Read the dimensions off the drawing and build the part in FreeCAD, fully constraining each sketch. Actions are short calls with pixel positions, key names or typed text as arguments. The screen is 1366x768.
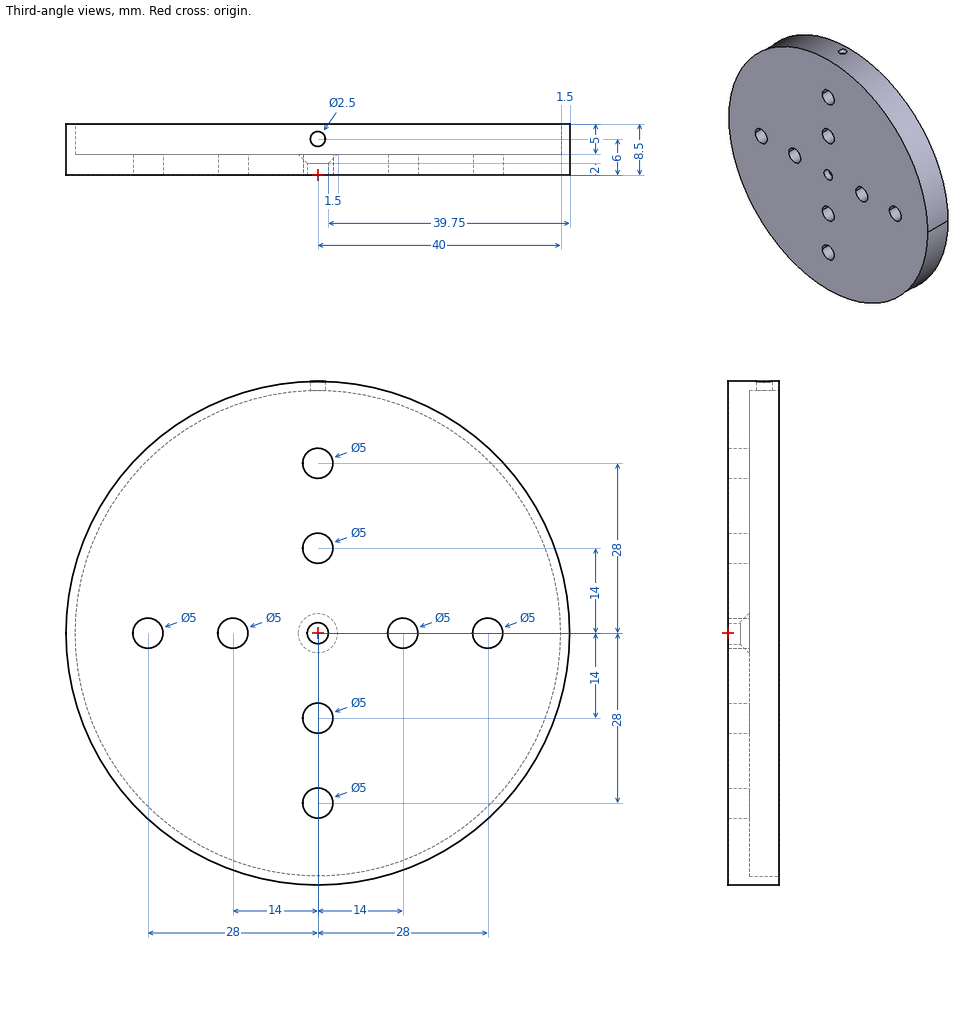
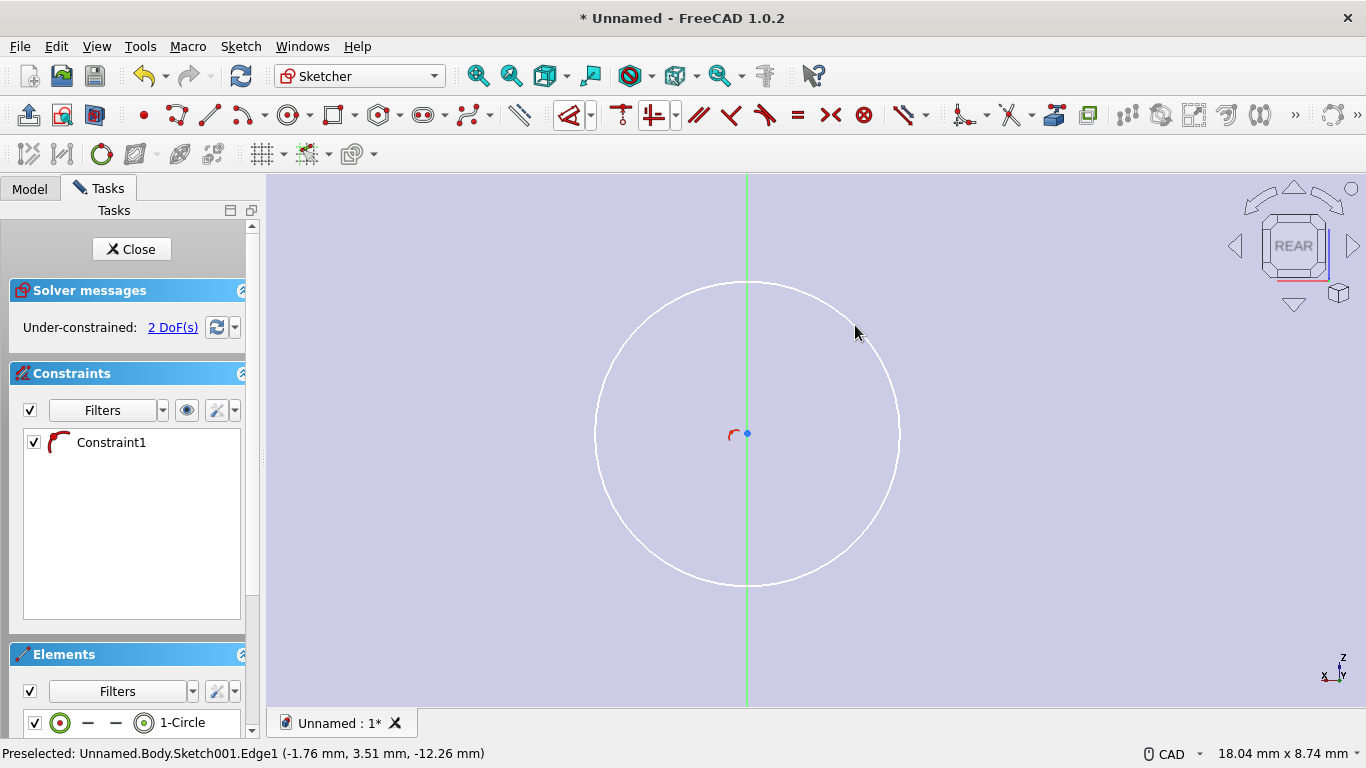
click(855, 326)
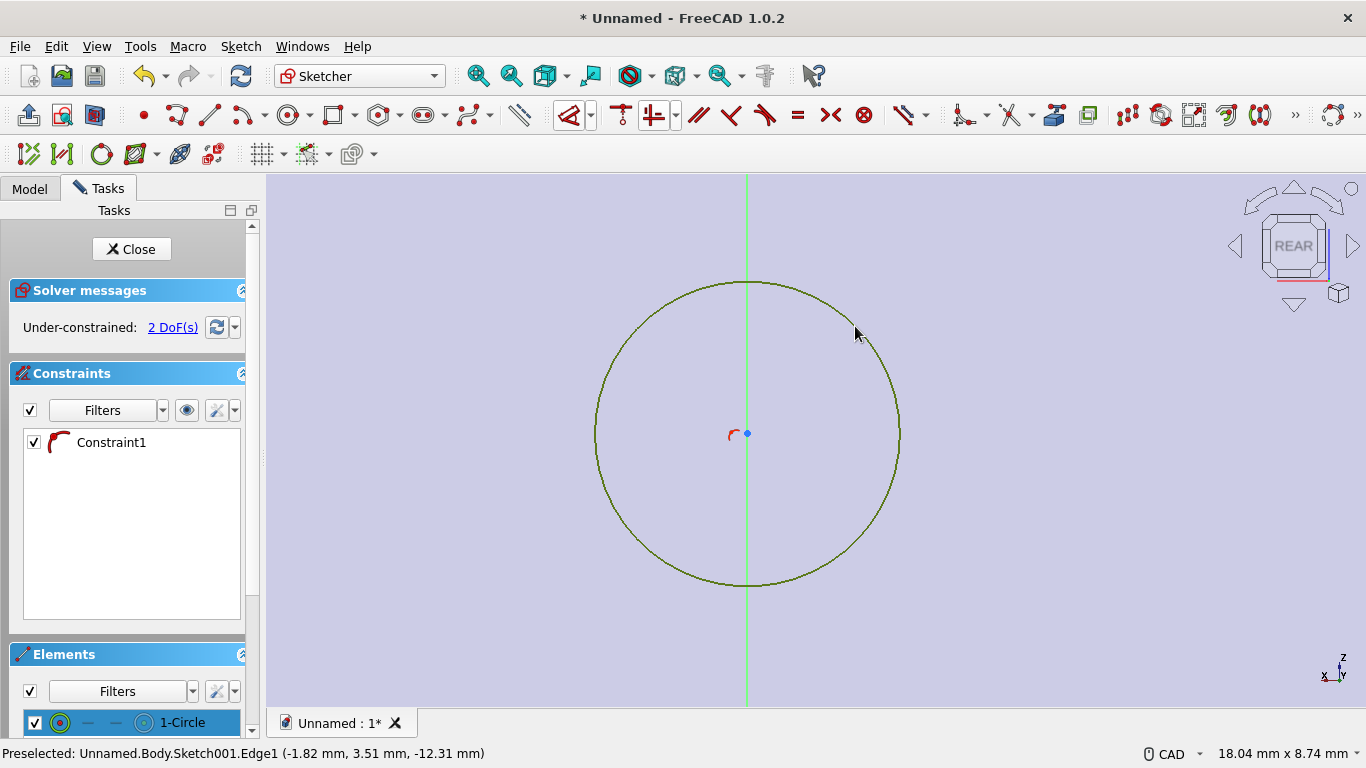
key(k)
key(o)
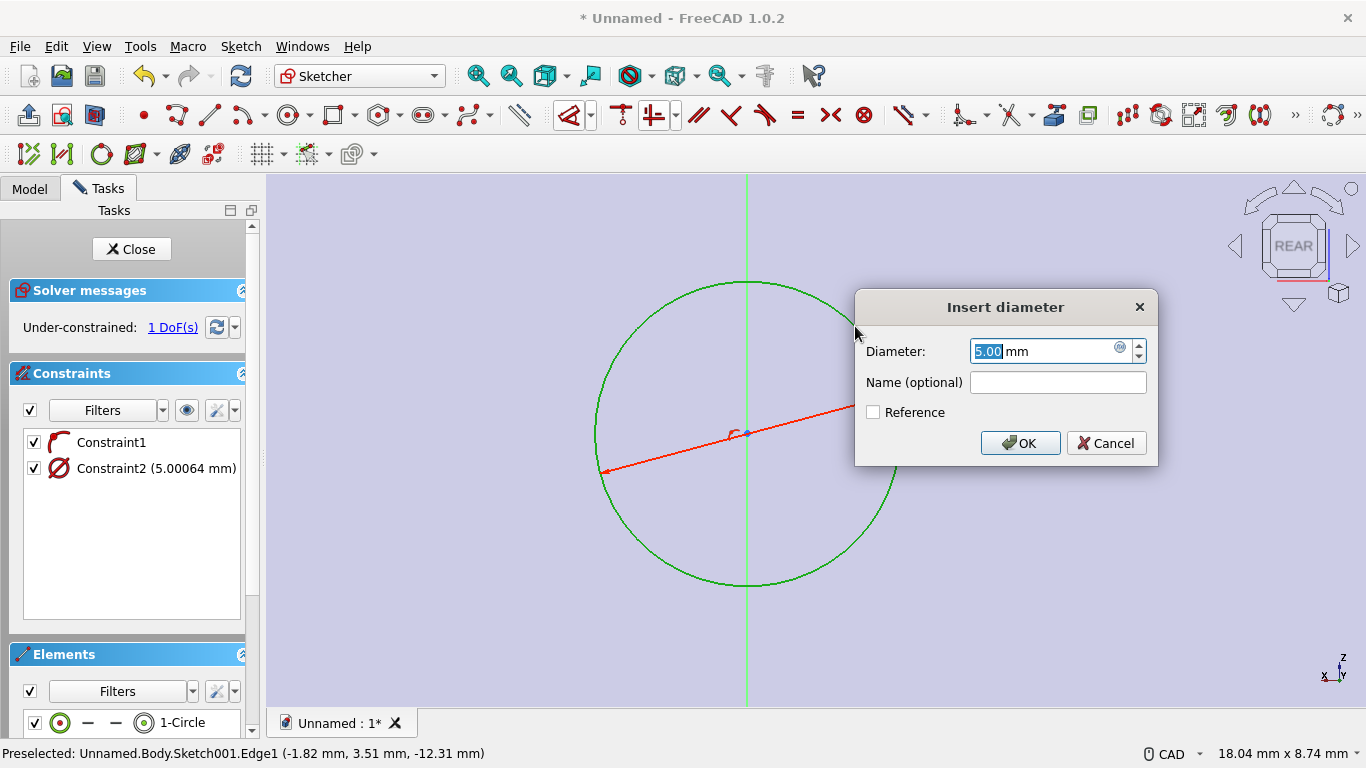
text(5)
key(Return)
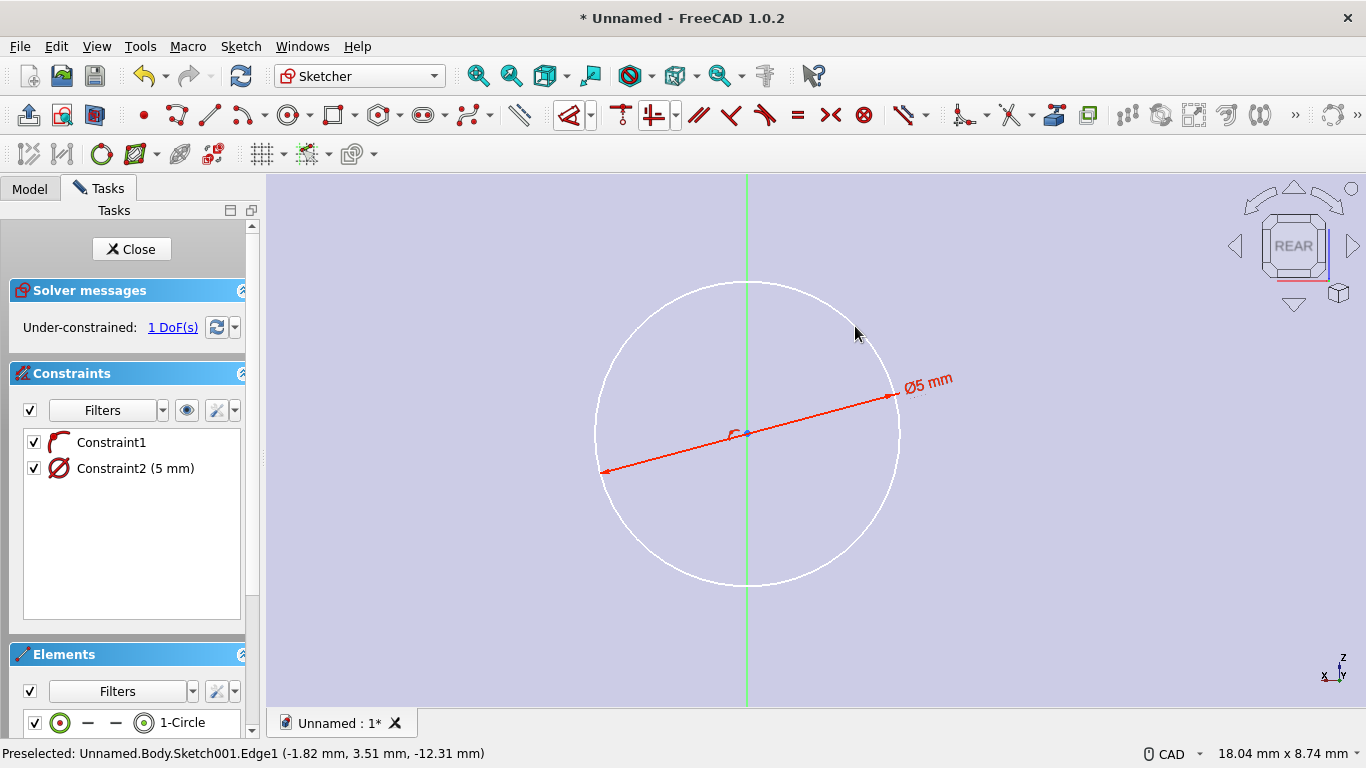
click(747, 434)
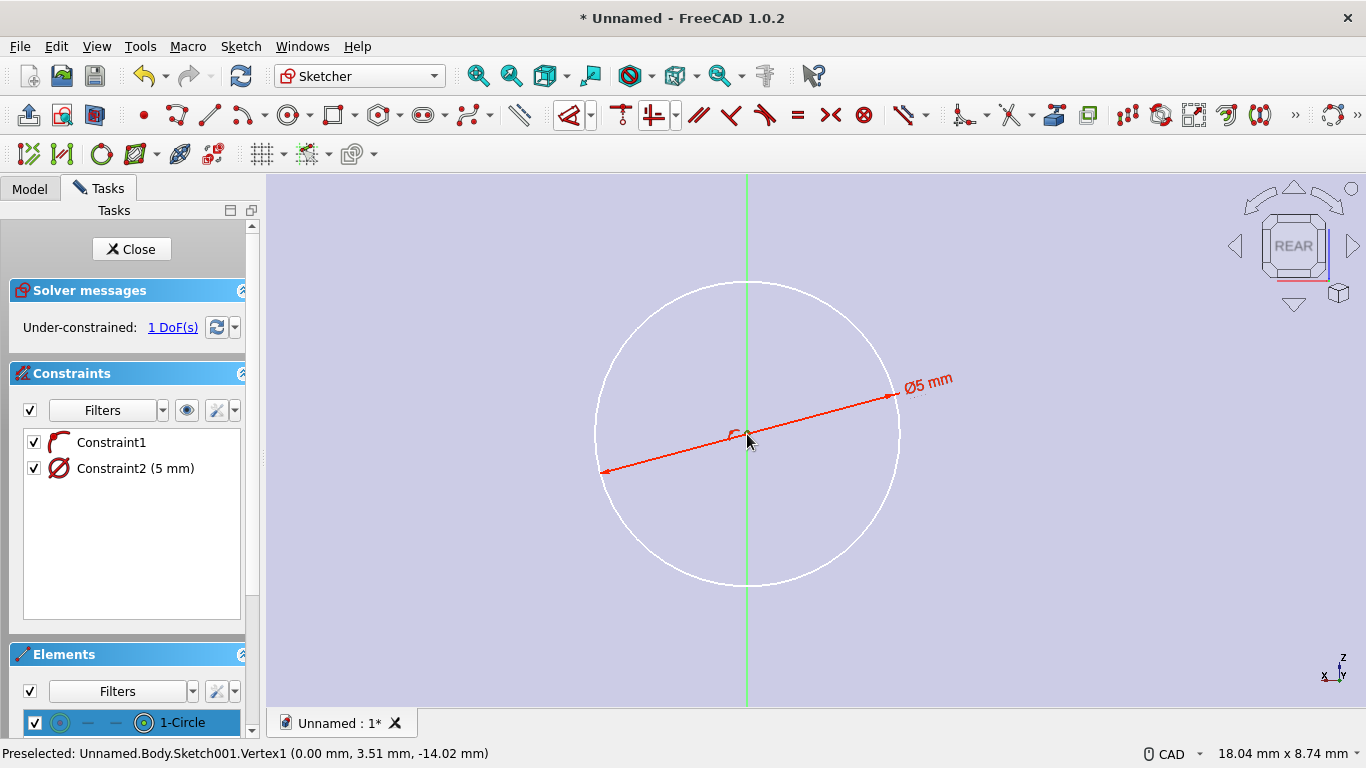
click(590, 116)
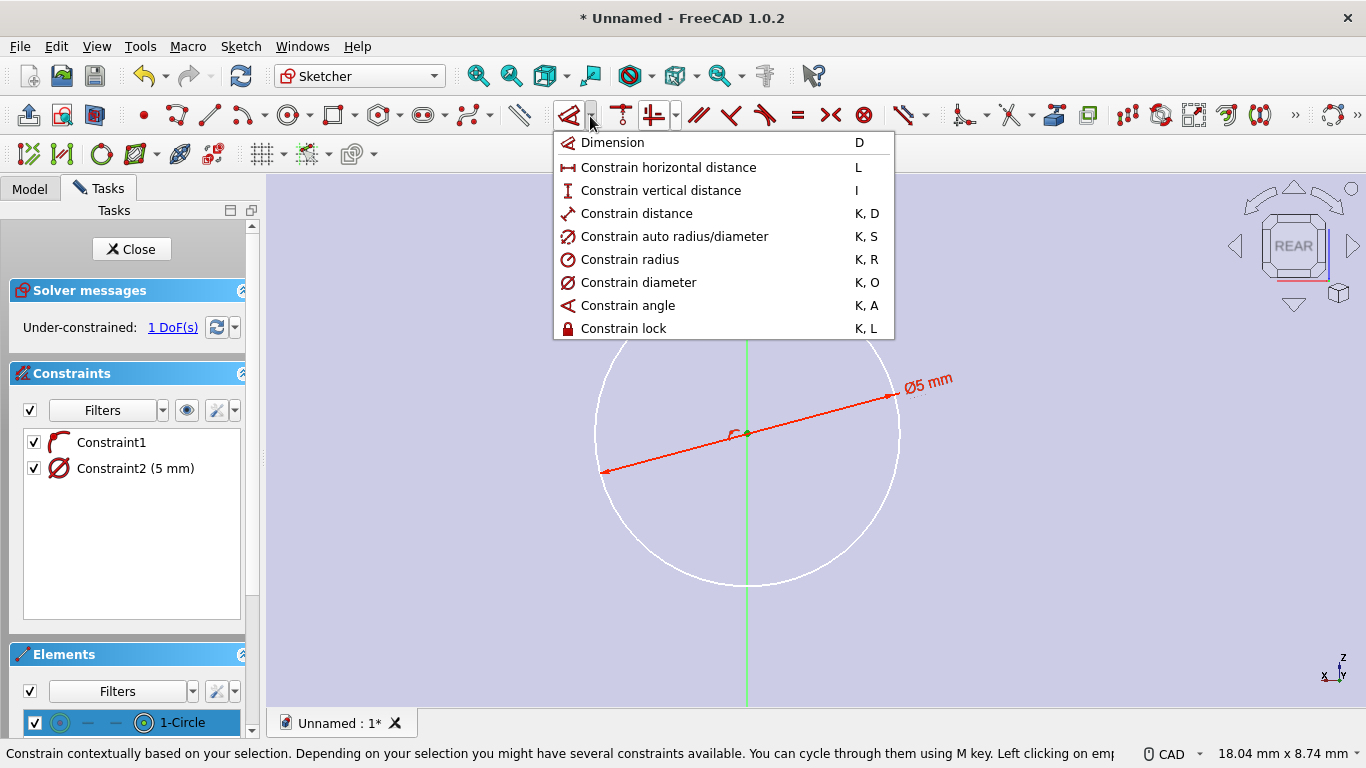
click(724, 190)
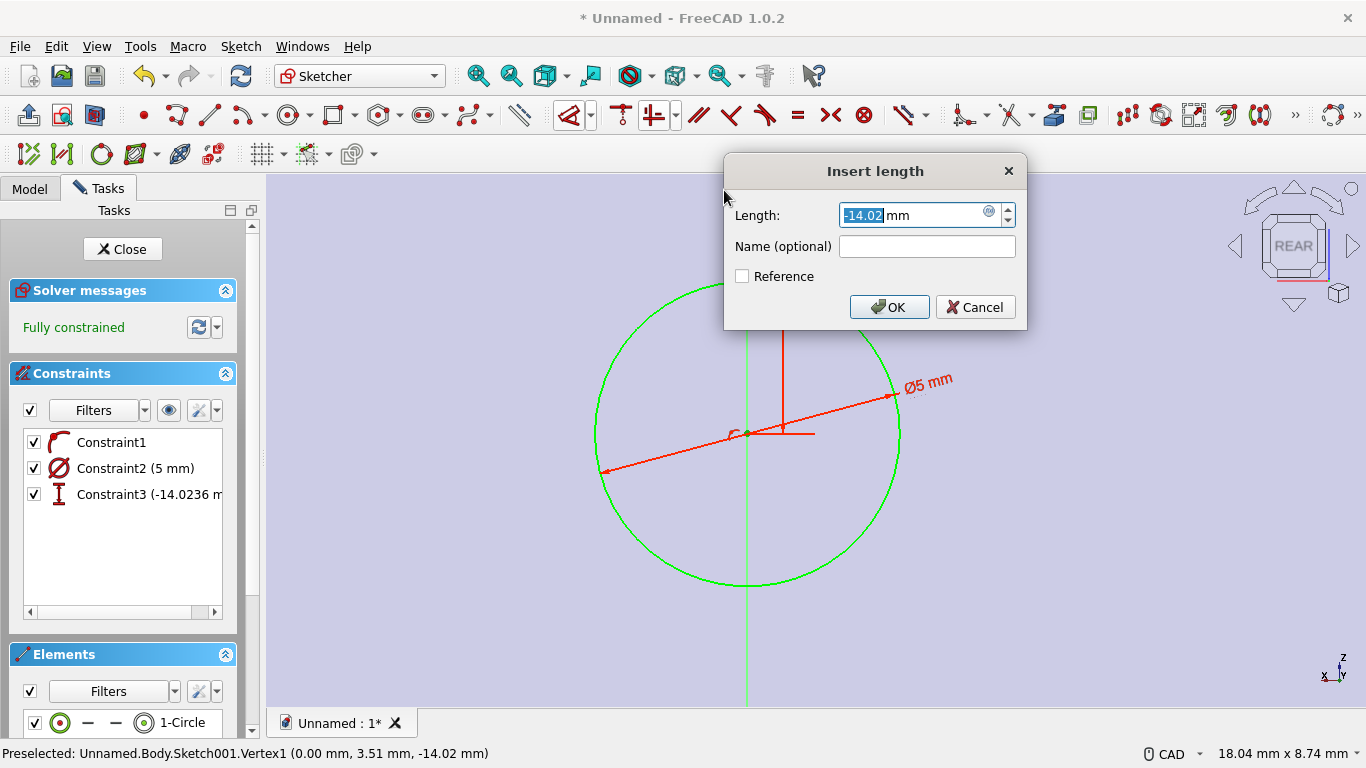
text(-14)
key(Return)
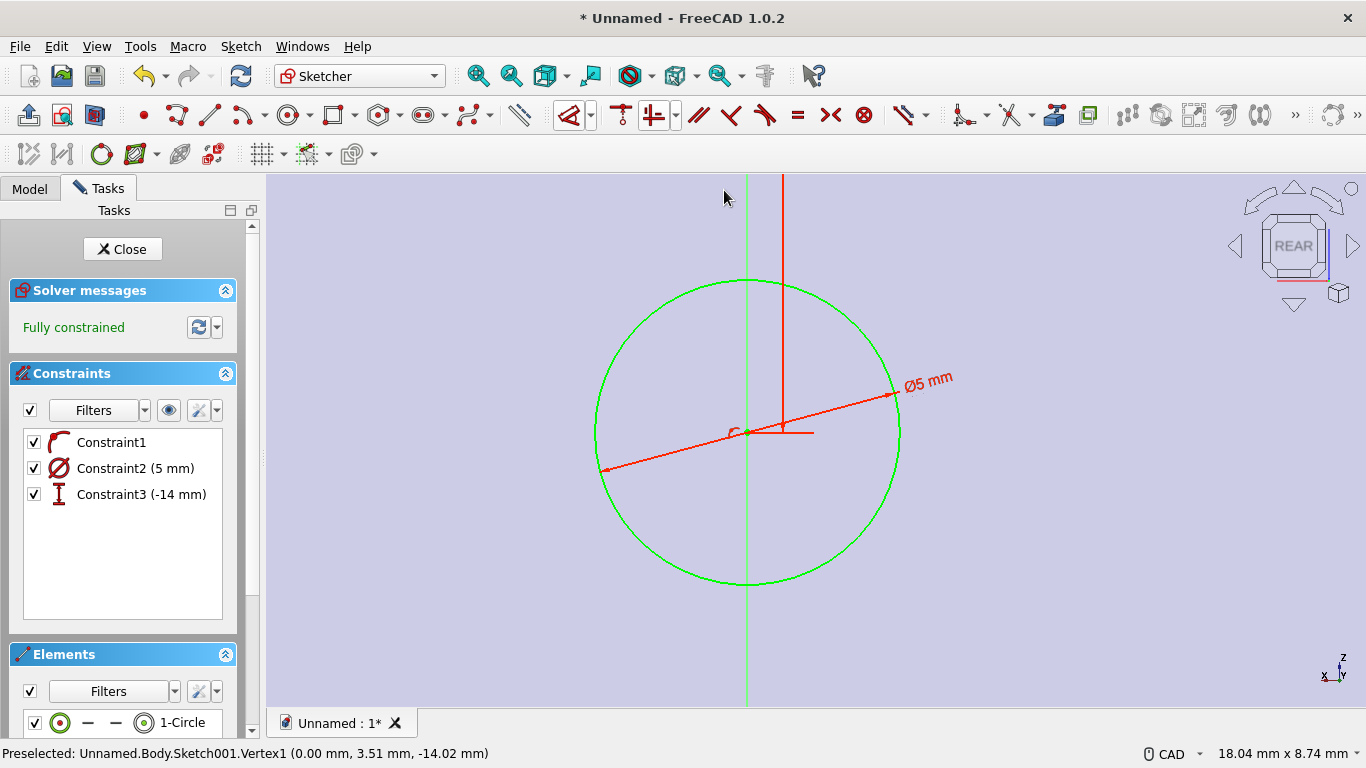
click(123, 249)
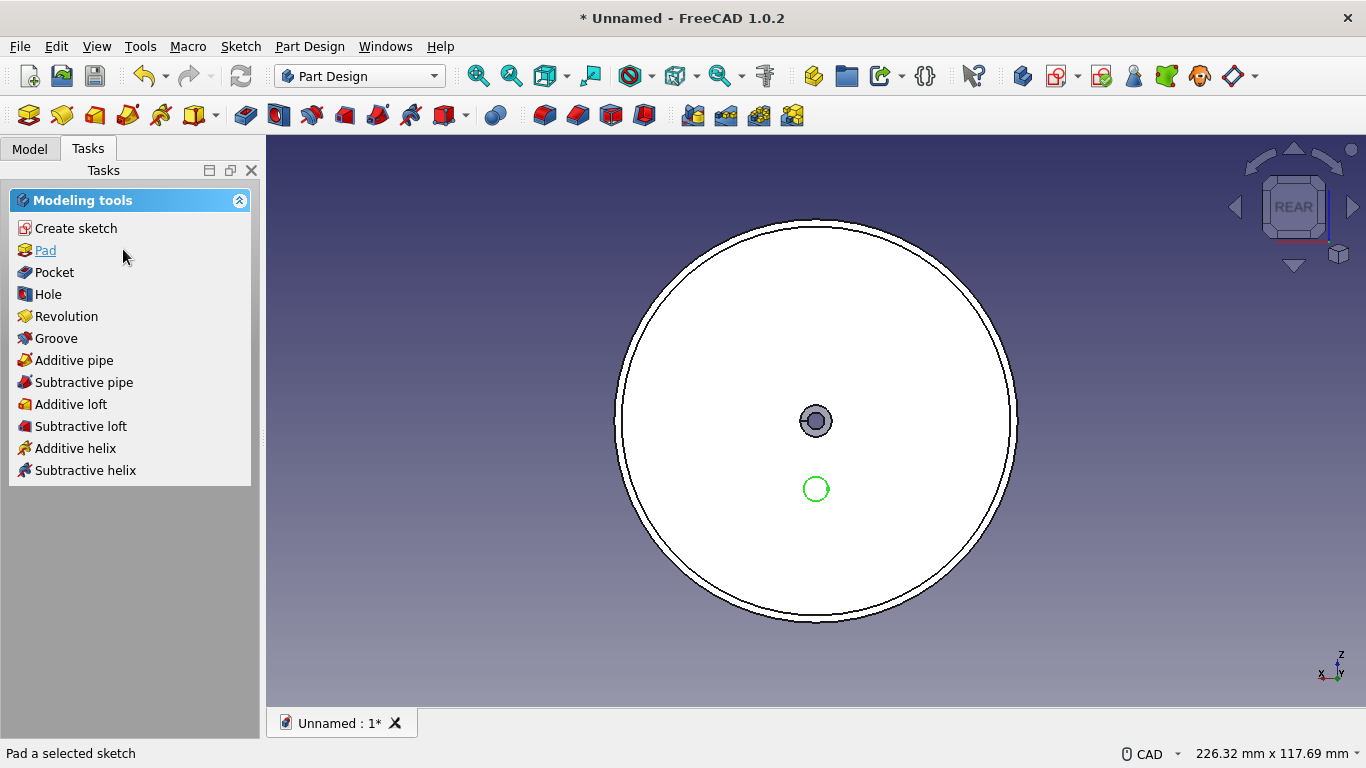
click(246, 116)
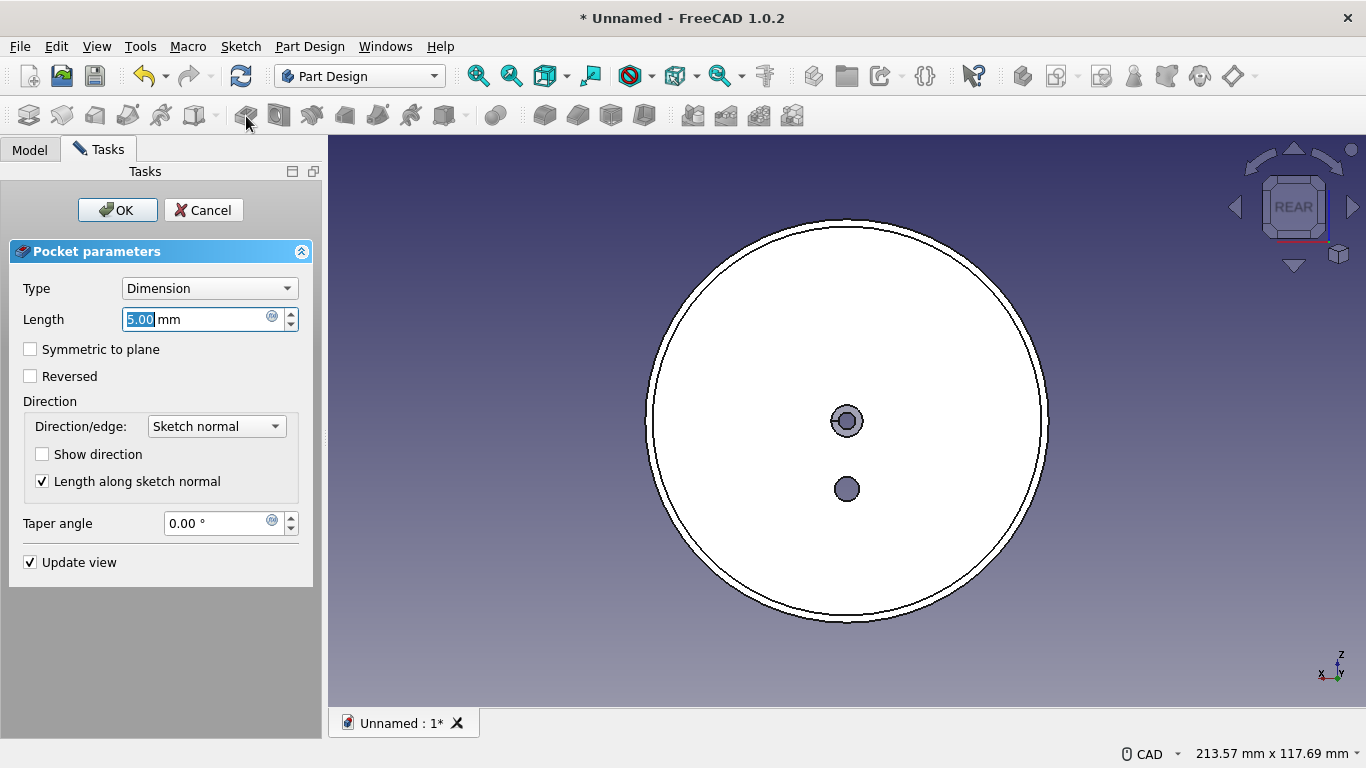
click(210, 288)